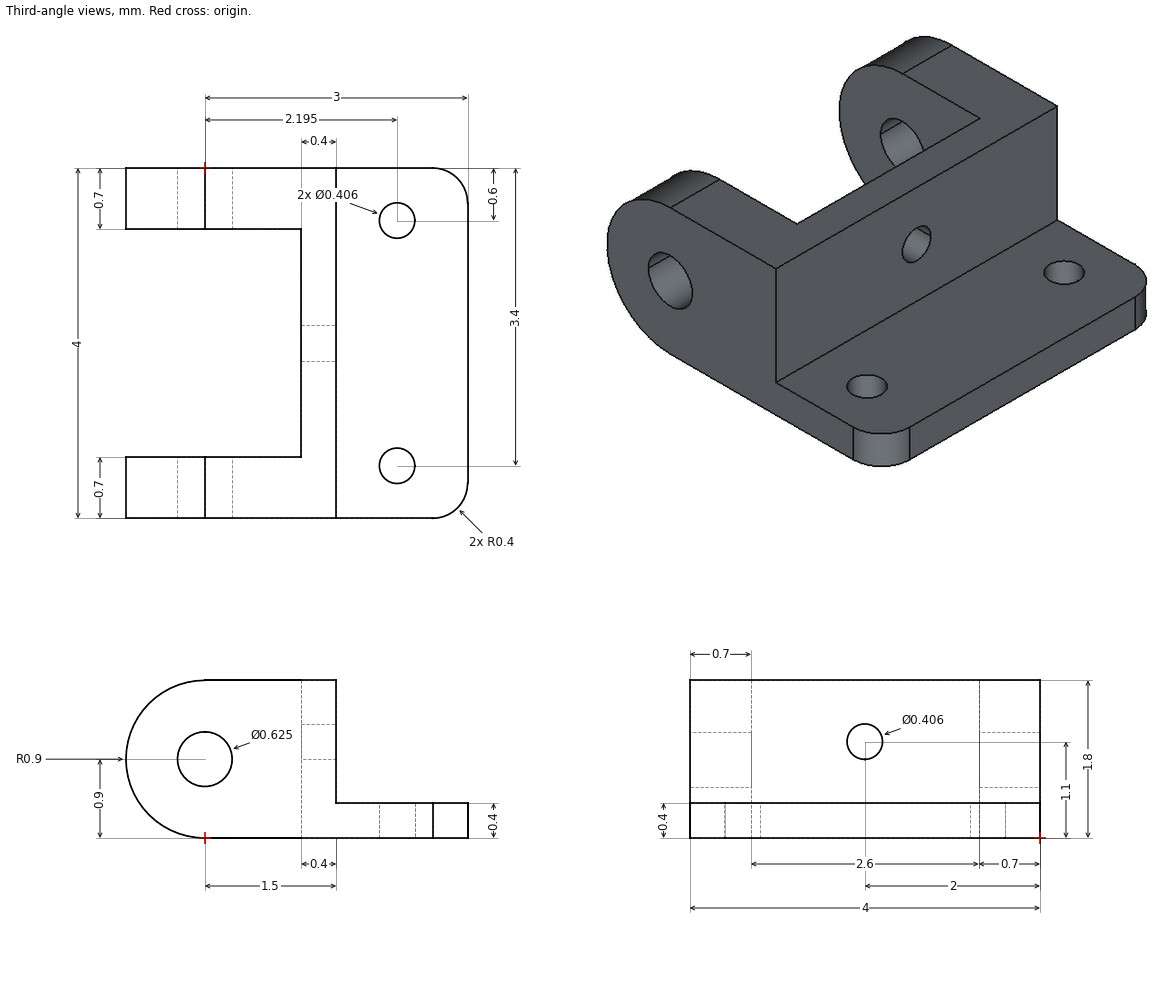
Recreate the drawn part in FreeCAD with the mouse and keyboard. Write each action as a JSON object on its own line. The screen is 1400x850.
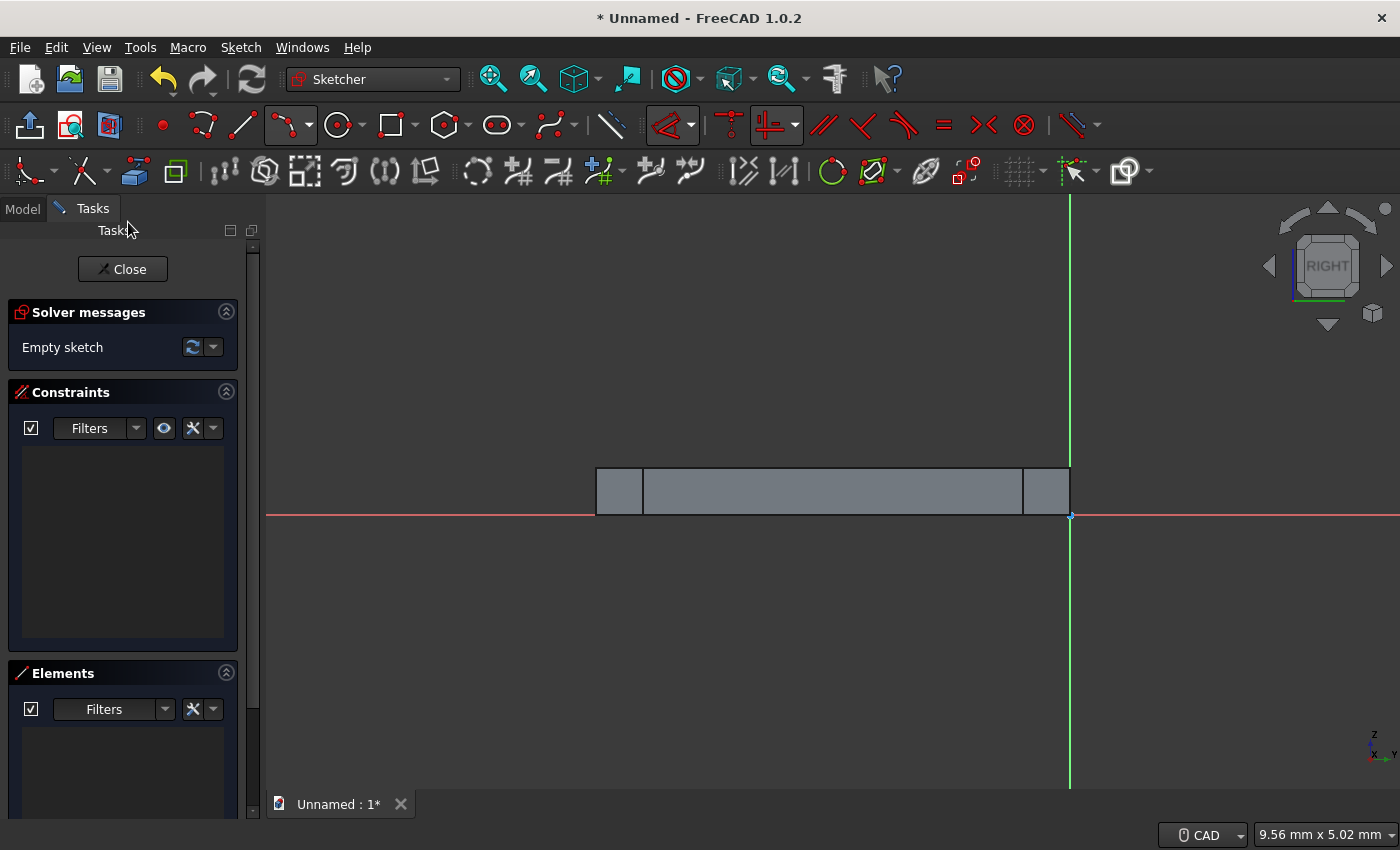
{"action": "key", "text": "q s"}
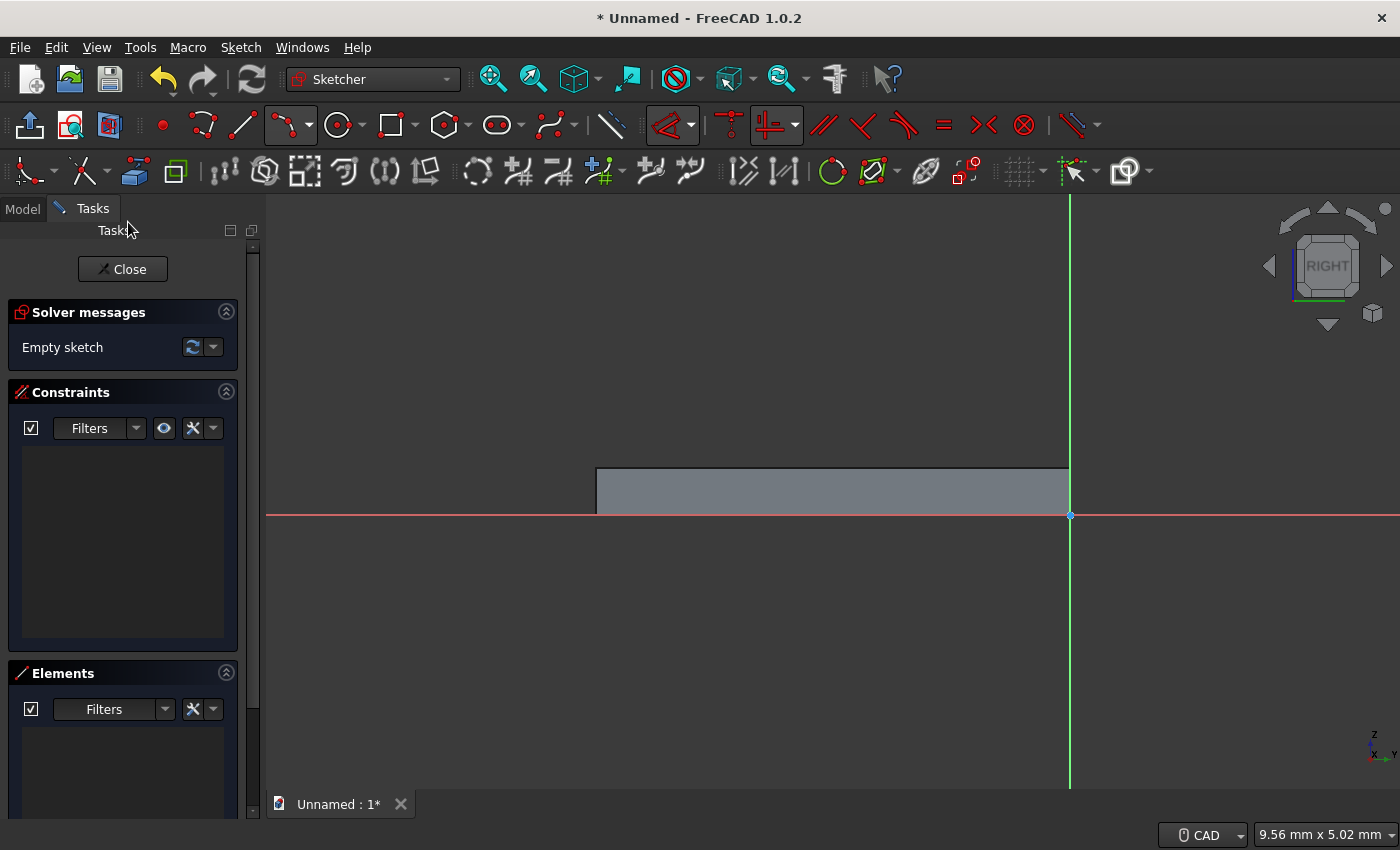
{"action": "scroll", "coordinate": [972, 492], "scroll_direction": "up", "scroll_amount": 2}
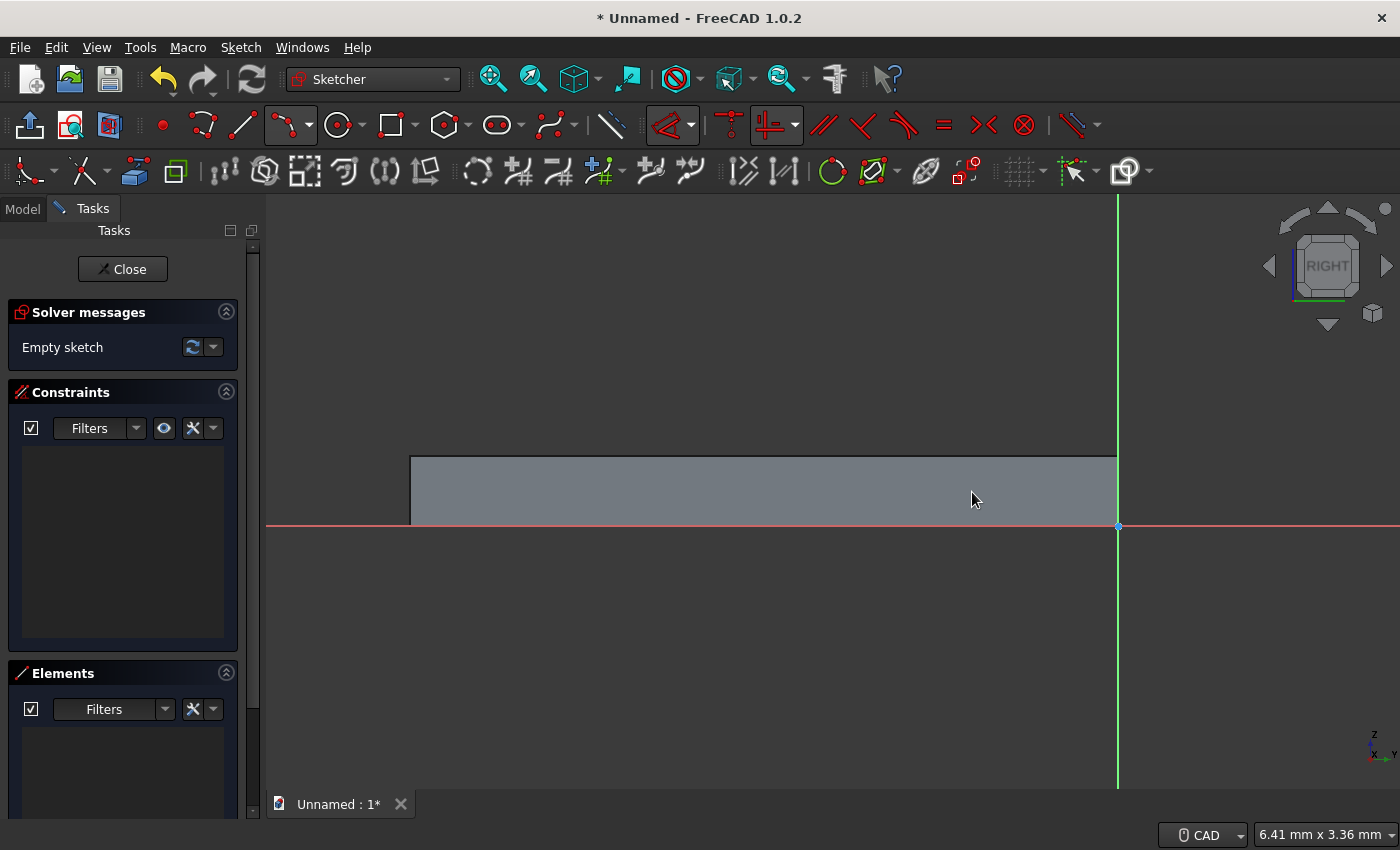
{"action": "key", "text": "g r"}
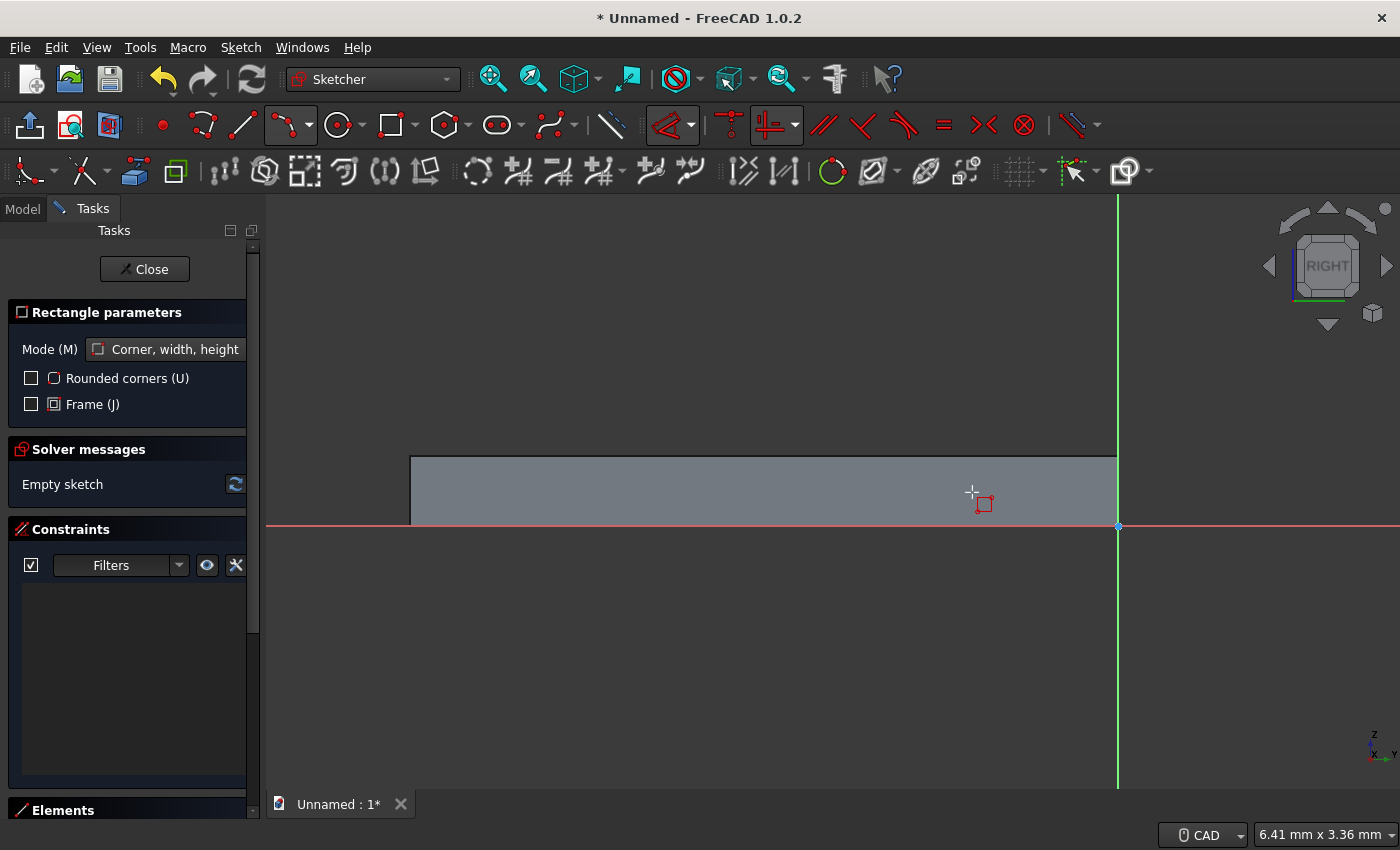
{"action": "left_click", "coordinate": [1118, 526]}
{"action": "mouse_move", "coordinate": [410, 456]}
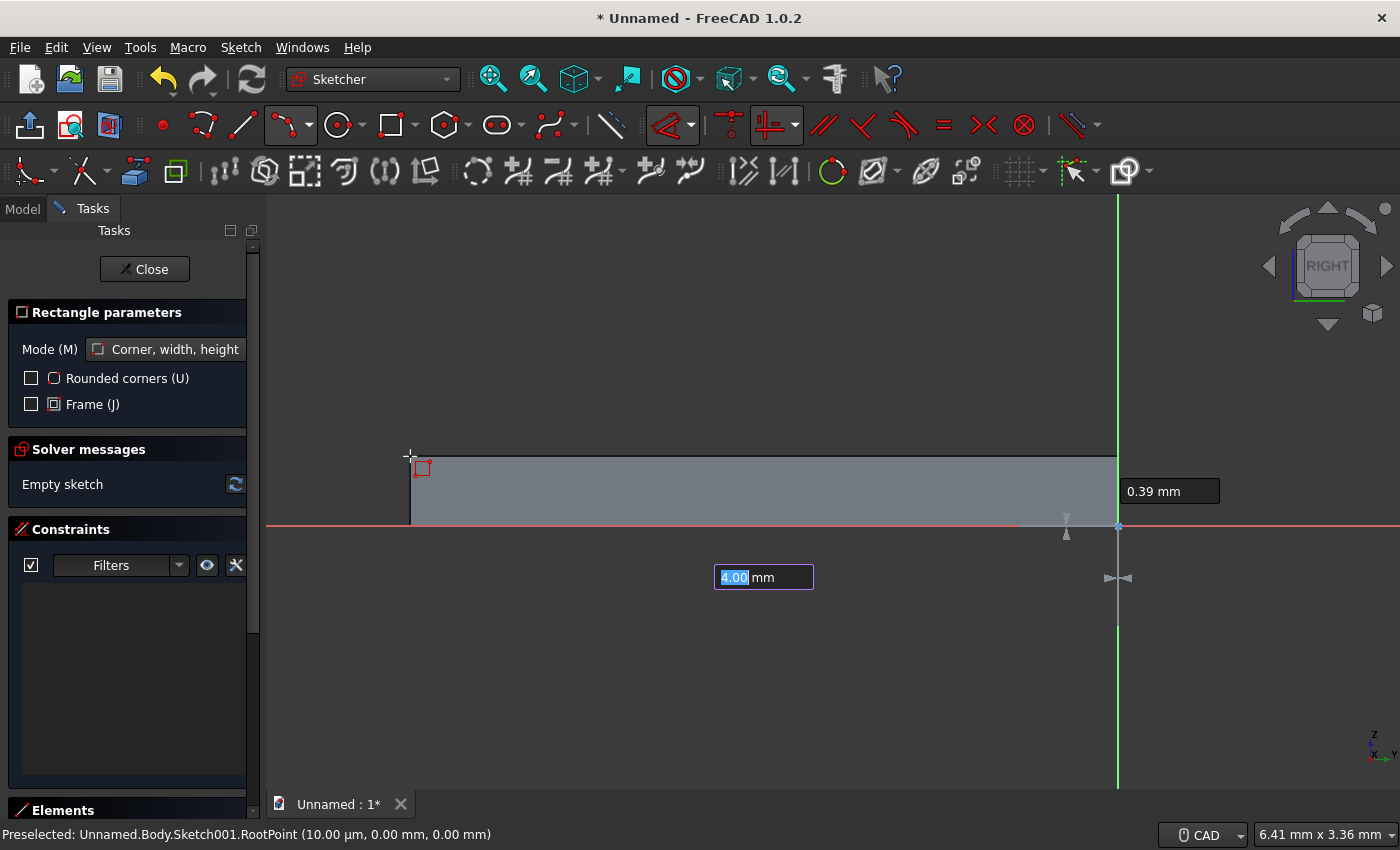
{"action": "type", "text": "4"}
{"action": "key", "text": "Tab"}
{"action": "type", "text": "0.4"}
{"action": "key", "text": "Return"}
{"action": "key", "text": "Escape"}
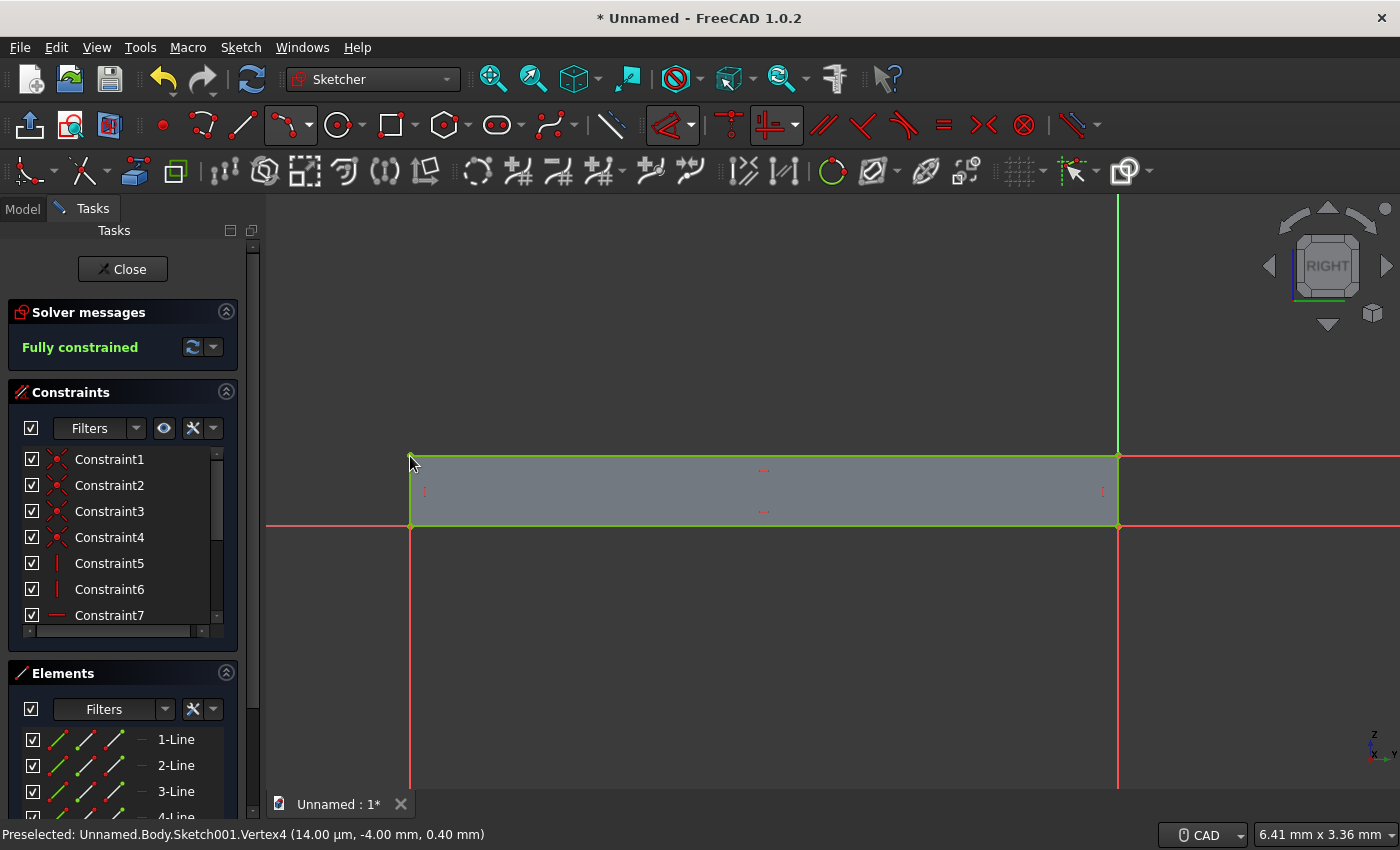
{"action": "left_click", "coordinate": [123, 269]}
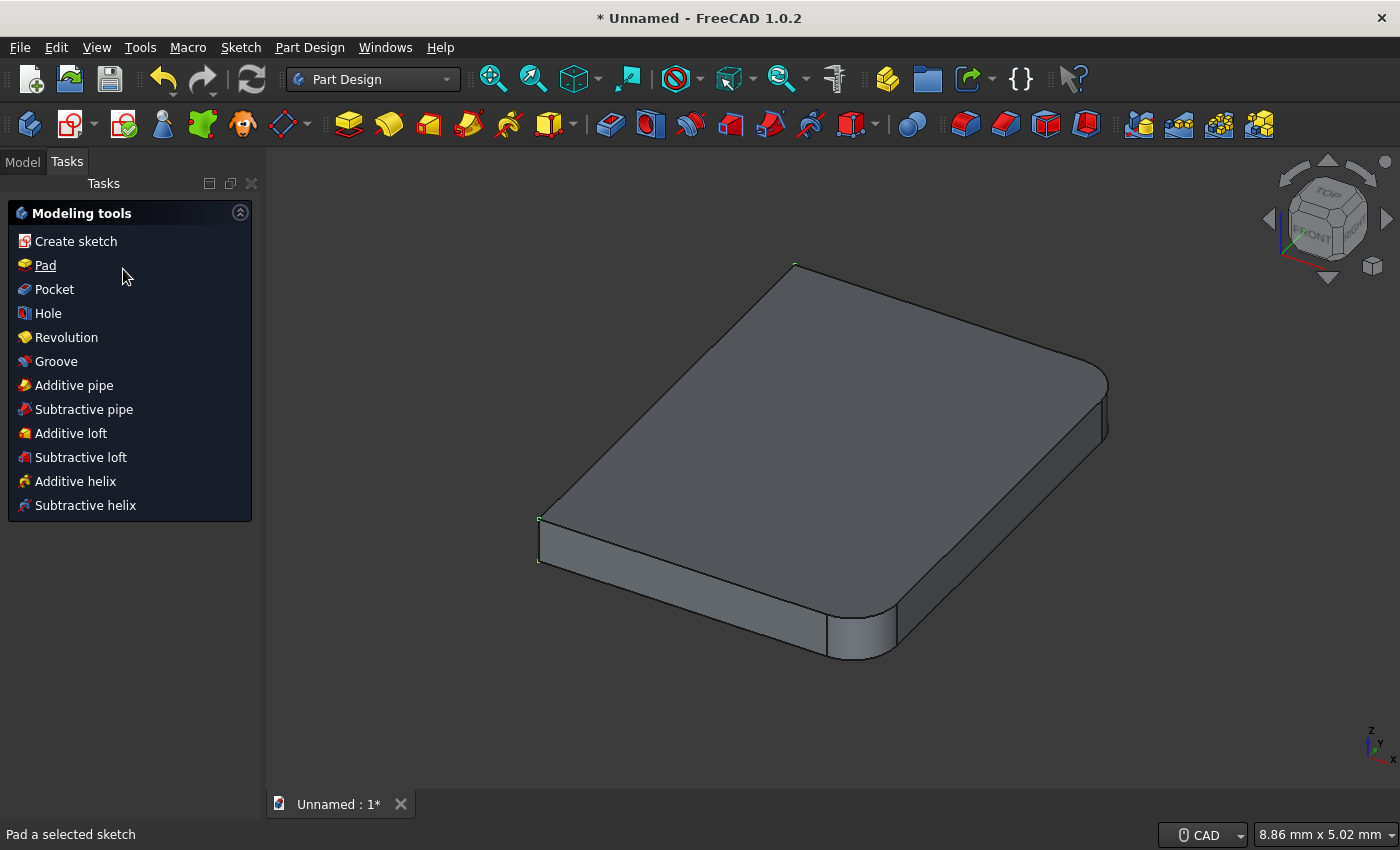
{"action": "left_click", "coordinate": [612, 124]}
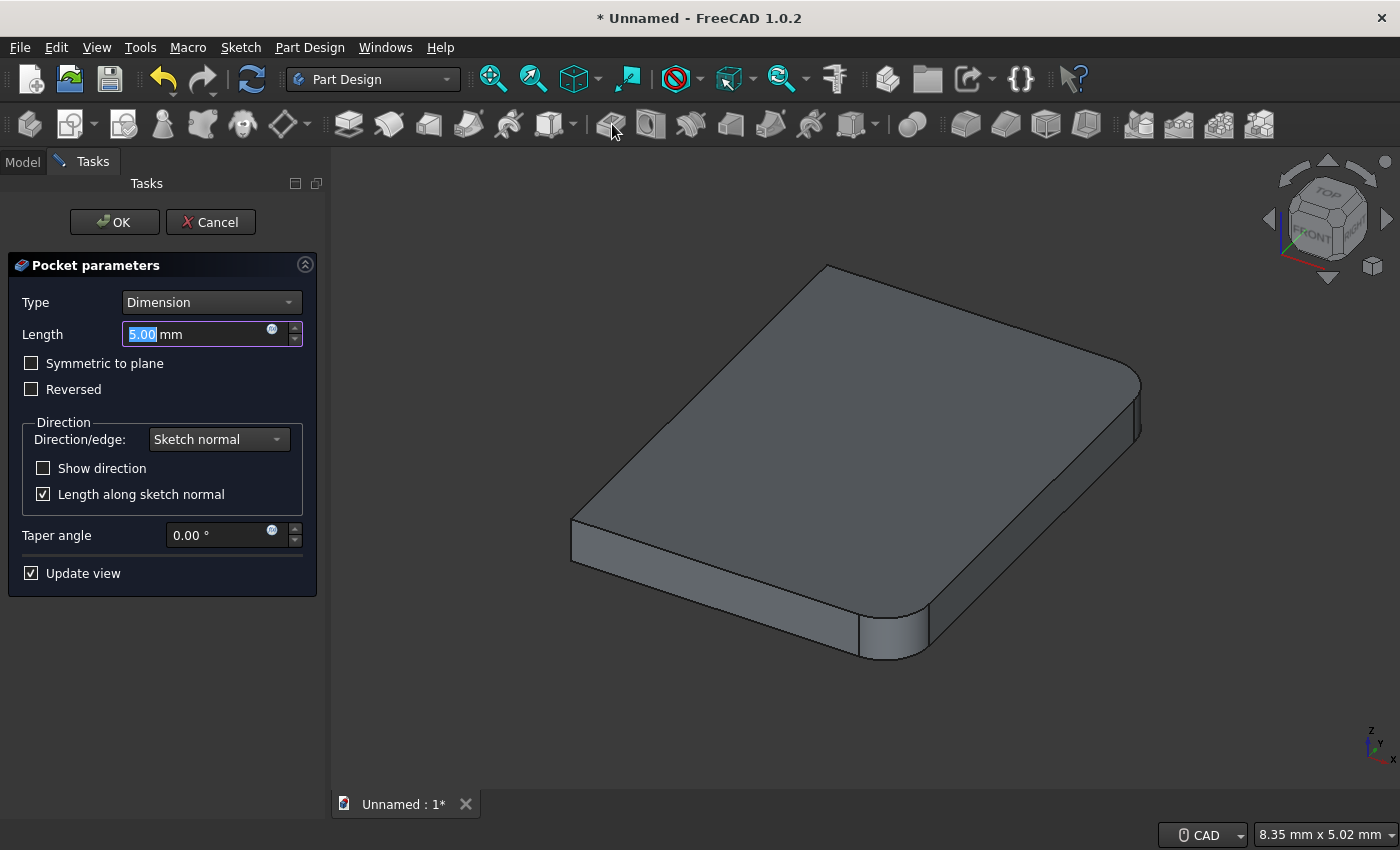
{"action": "type", "text": "1.5"}
{"action": "key", "text": "Tab"}